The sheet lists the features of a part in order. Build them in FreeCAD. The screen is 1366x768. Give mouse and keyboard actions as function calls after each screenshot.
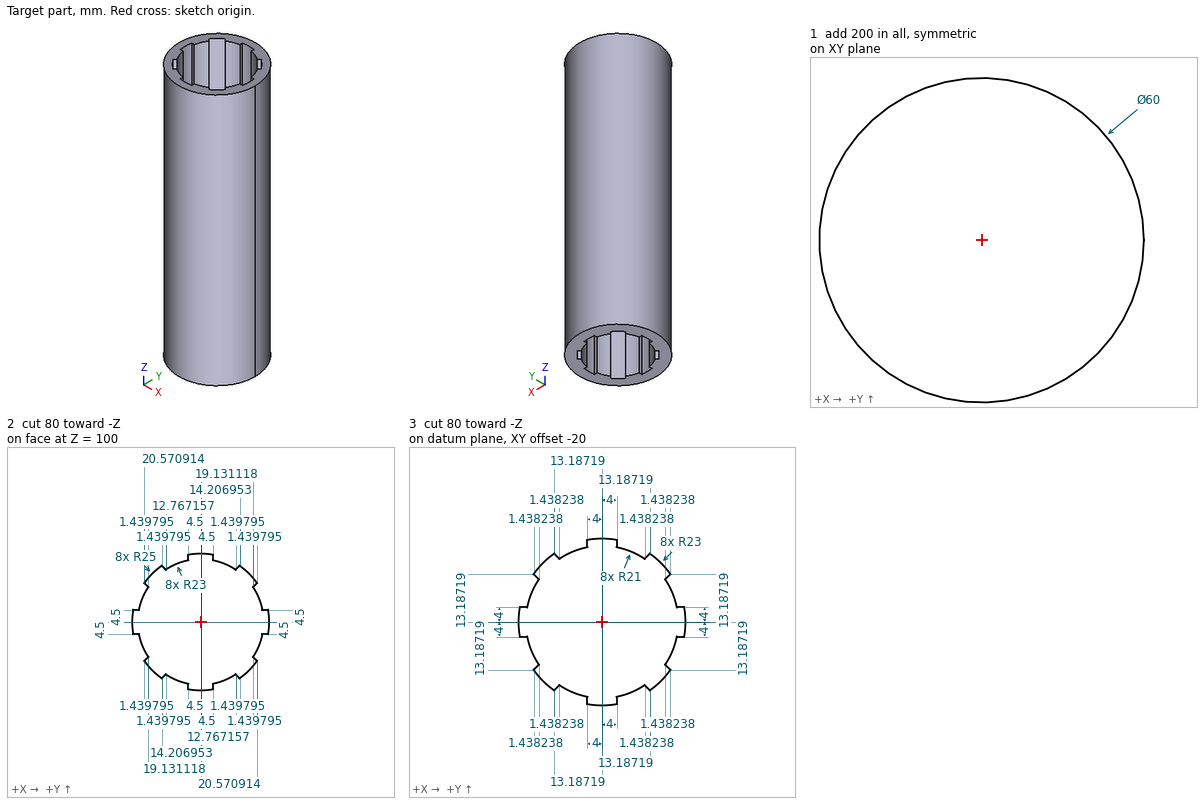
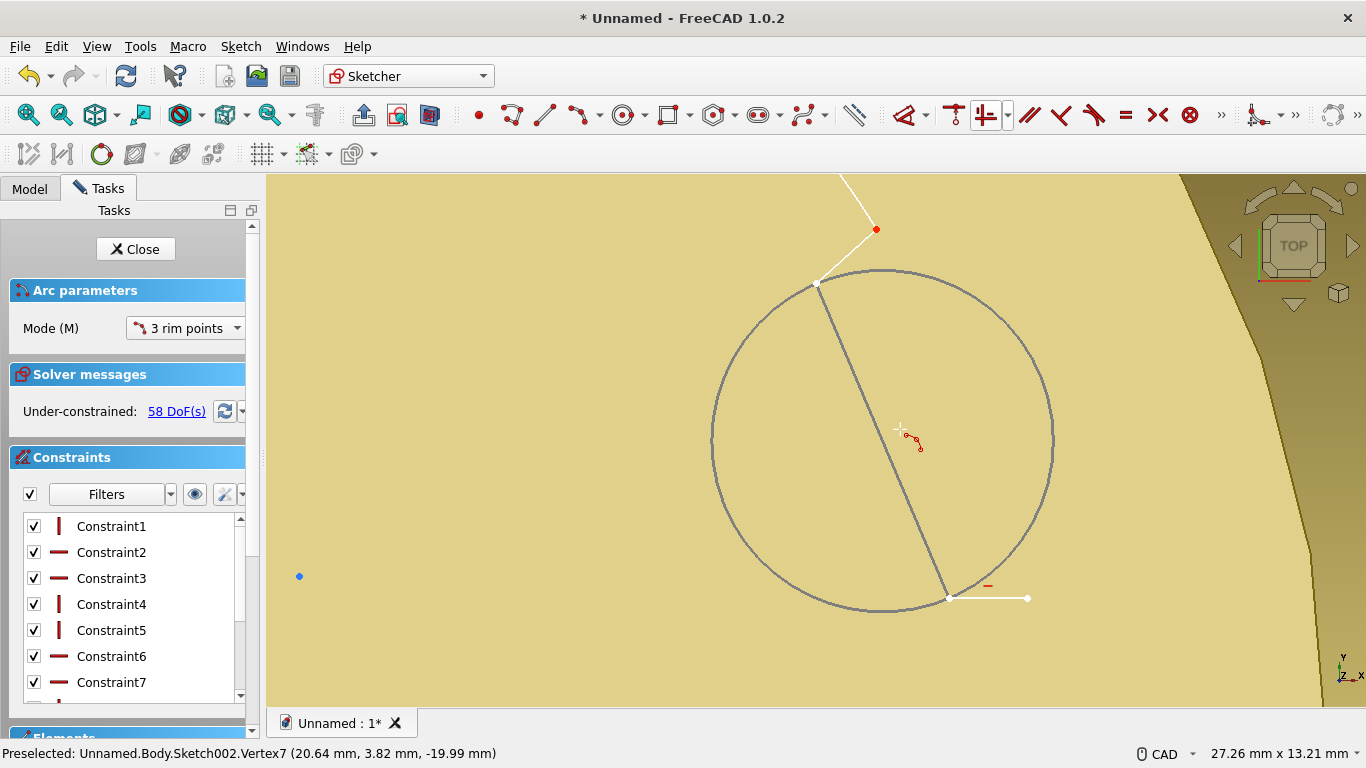
click(899, 428)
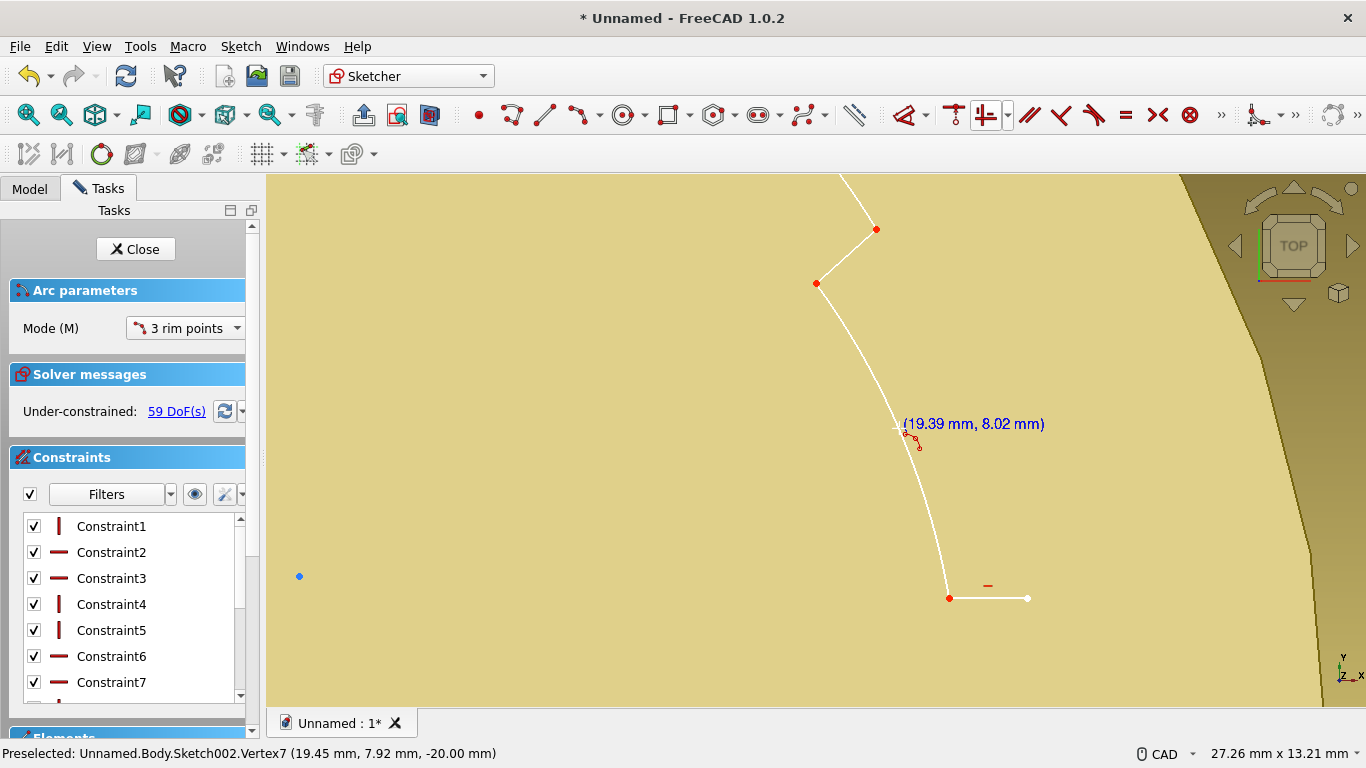
click(1028, 598)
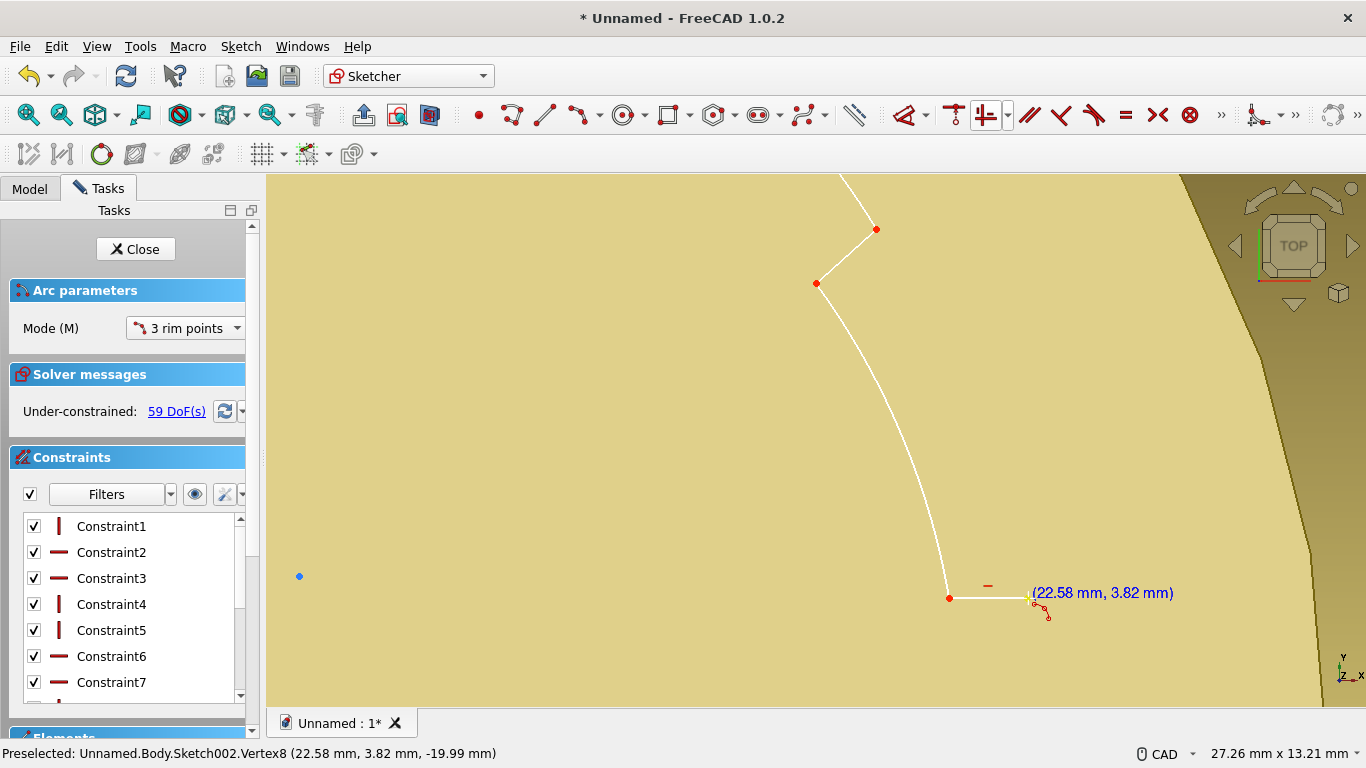
scroll(872, 379, down, 9)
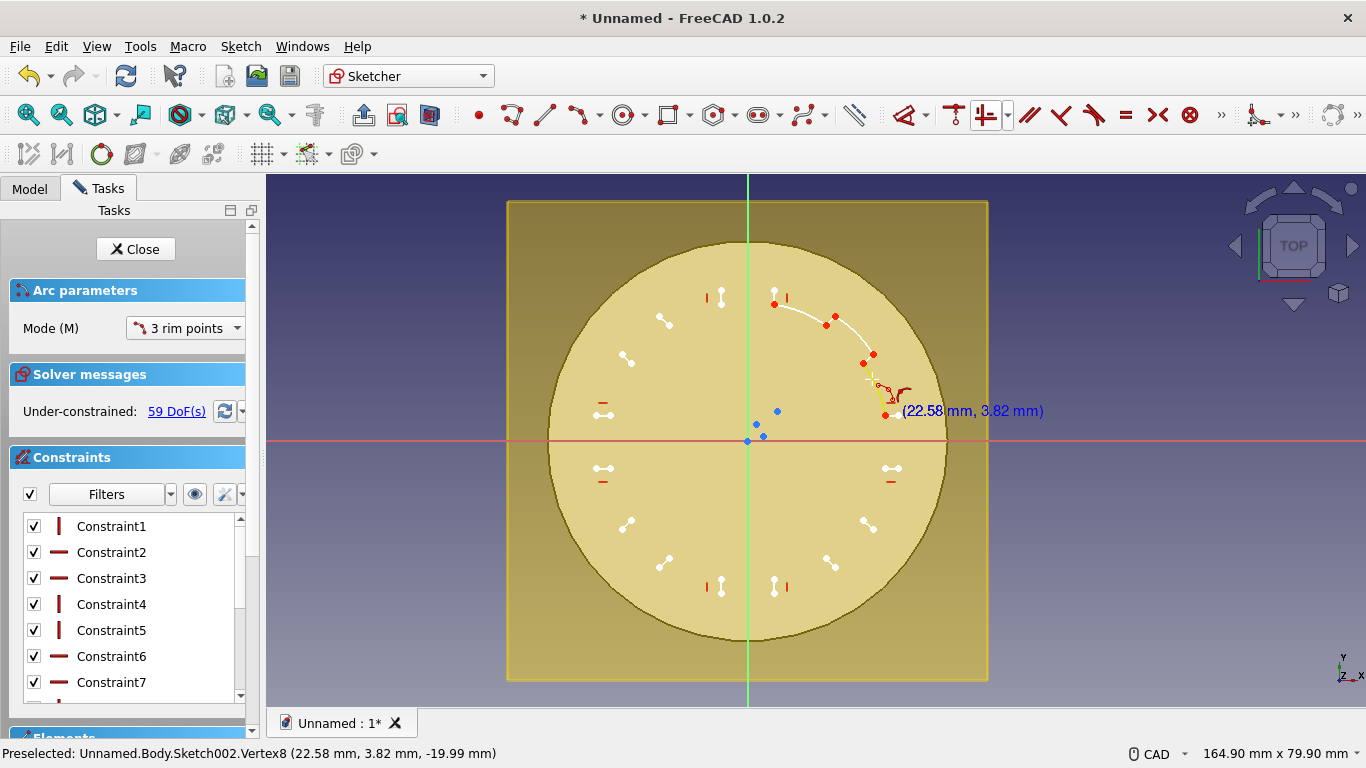
scroll(899, 468, up, 5)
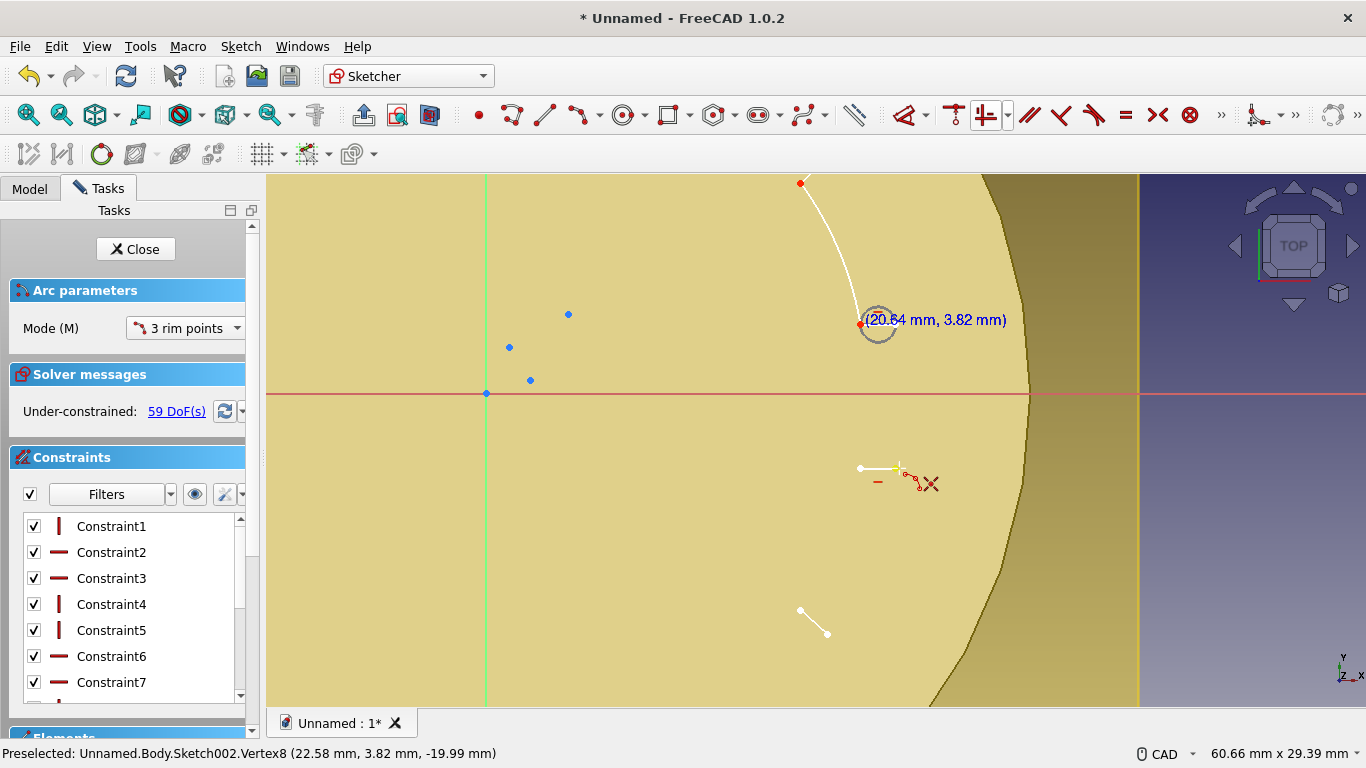
click(896, 469)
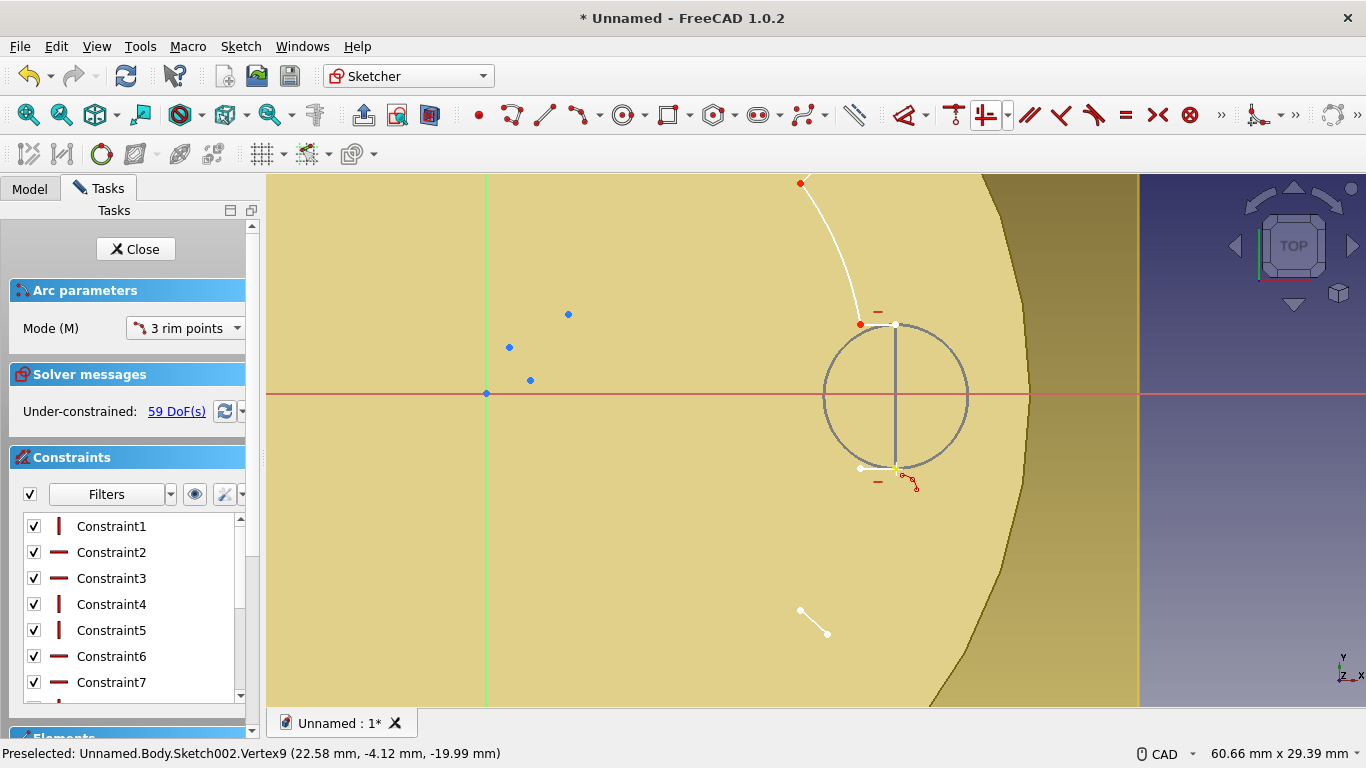
scroll(903, 408, up, 5)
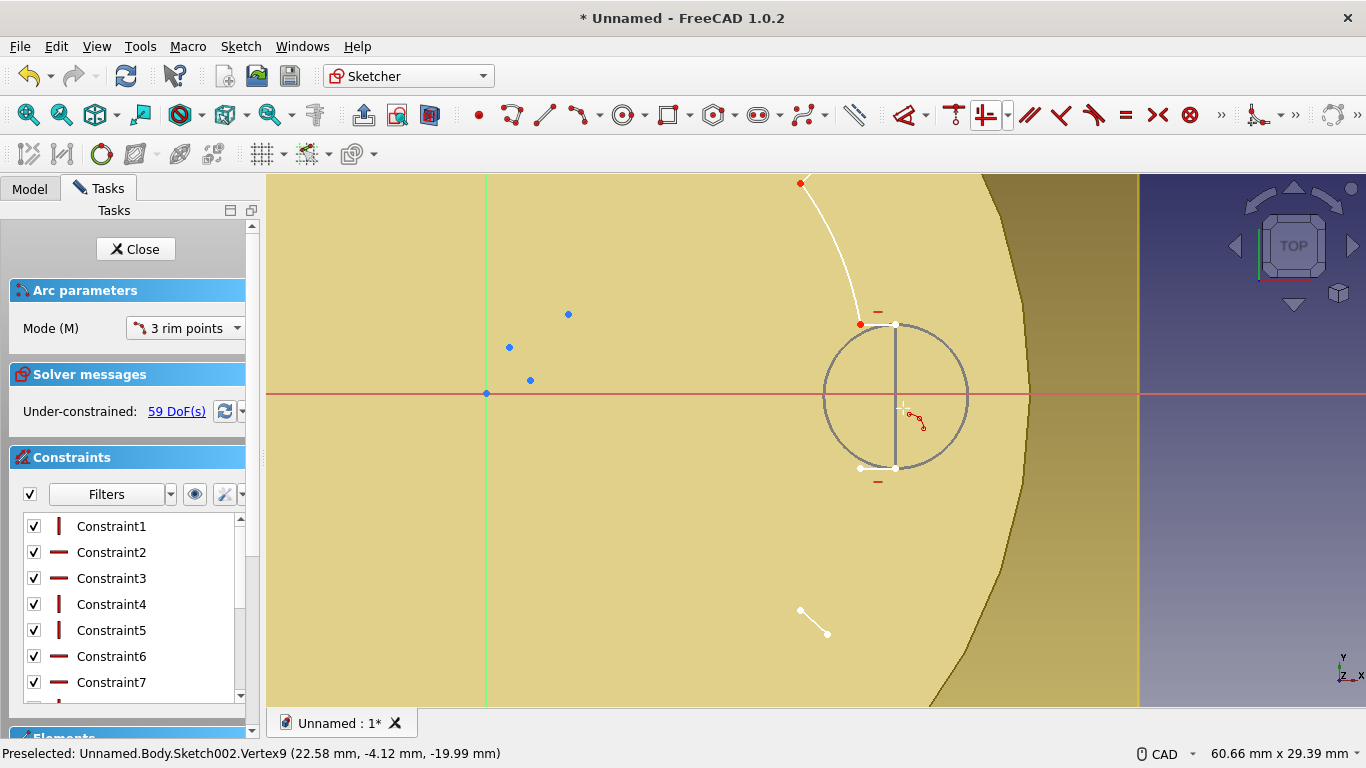
click(902, 409)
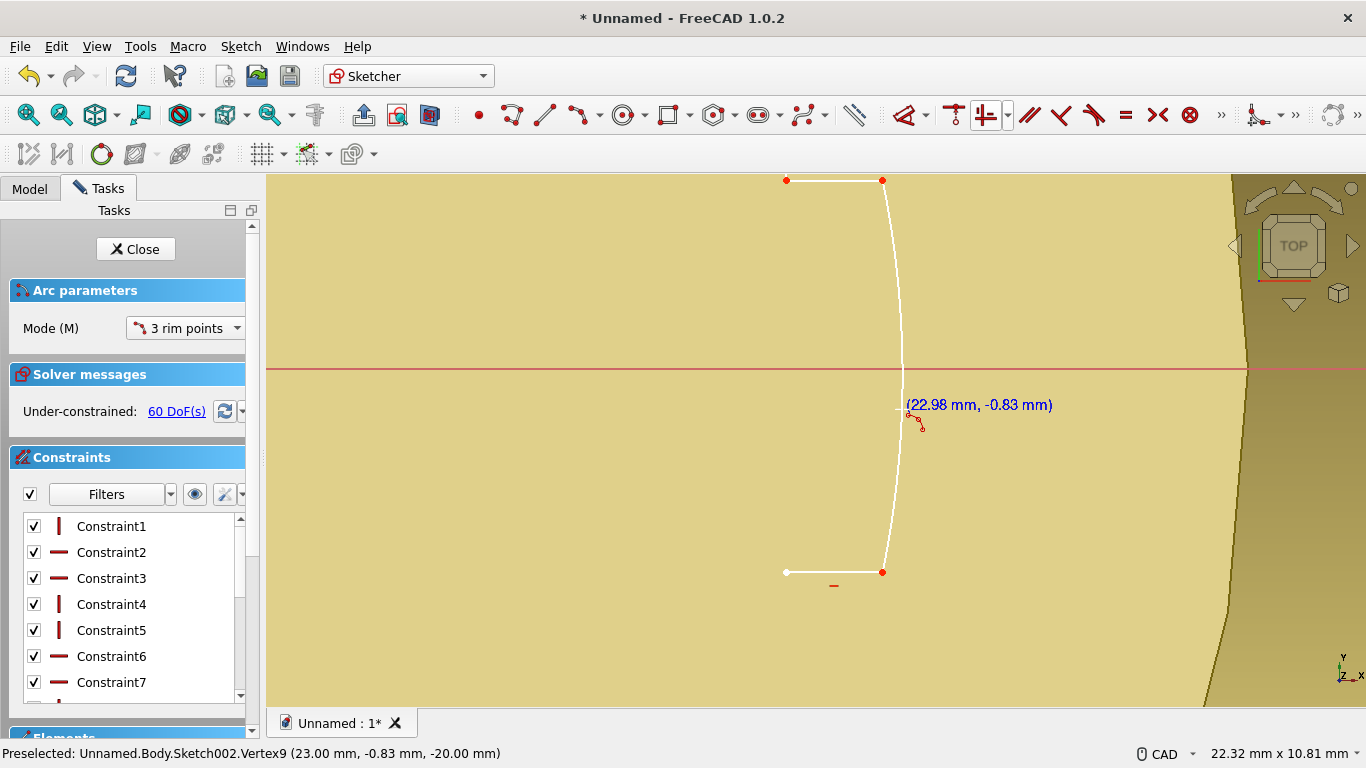
scroll(901, 452, down, 10)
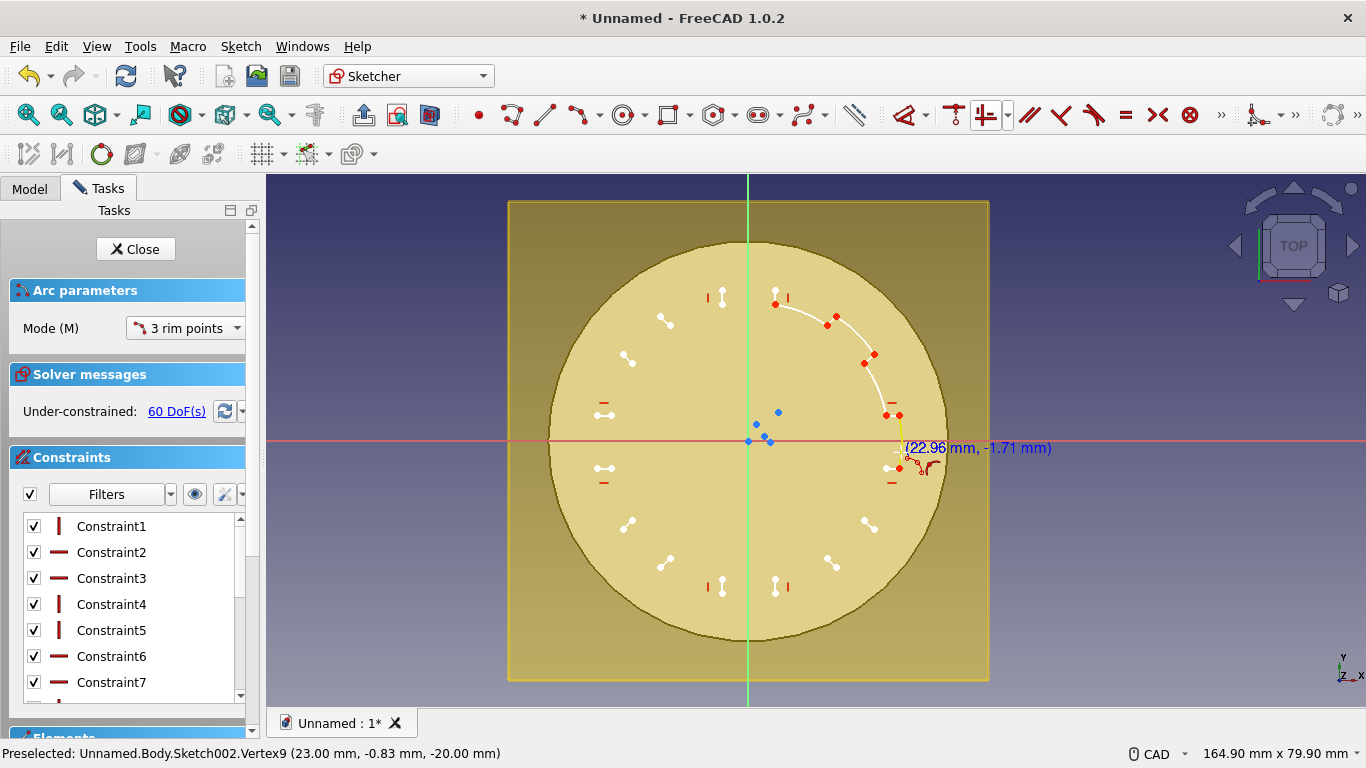
scroll(886, 468, up, 5)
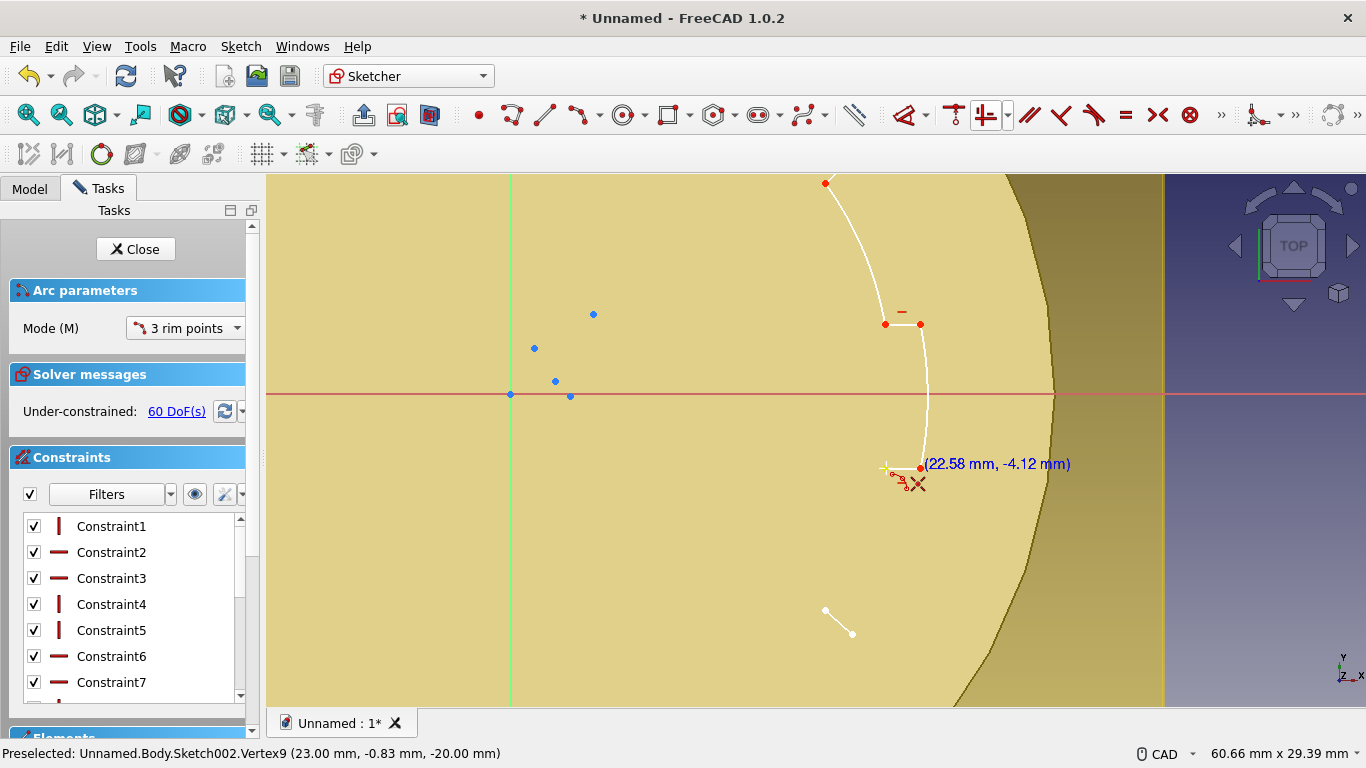
click(885, 469)
click(825, 610)